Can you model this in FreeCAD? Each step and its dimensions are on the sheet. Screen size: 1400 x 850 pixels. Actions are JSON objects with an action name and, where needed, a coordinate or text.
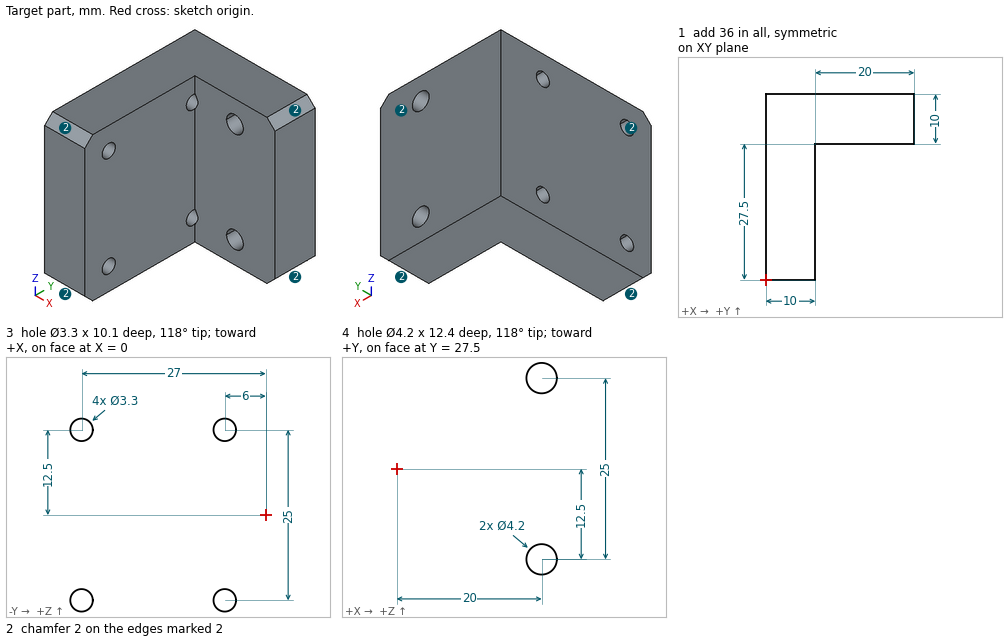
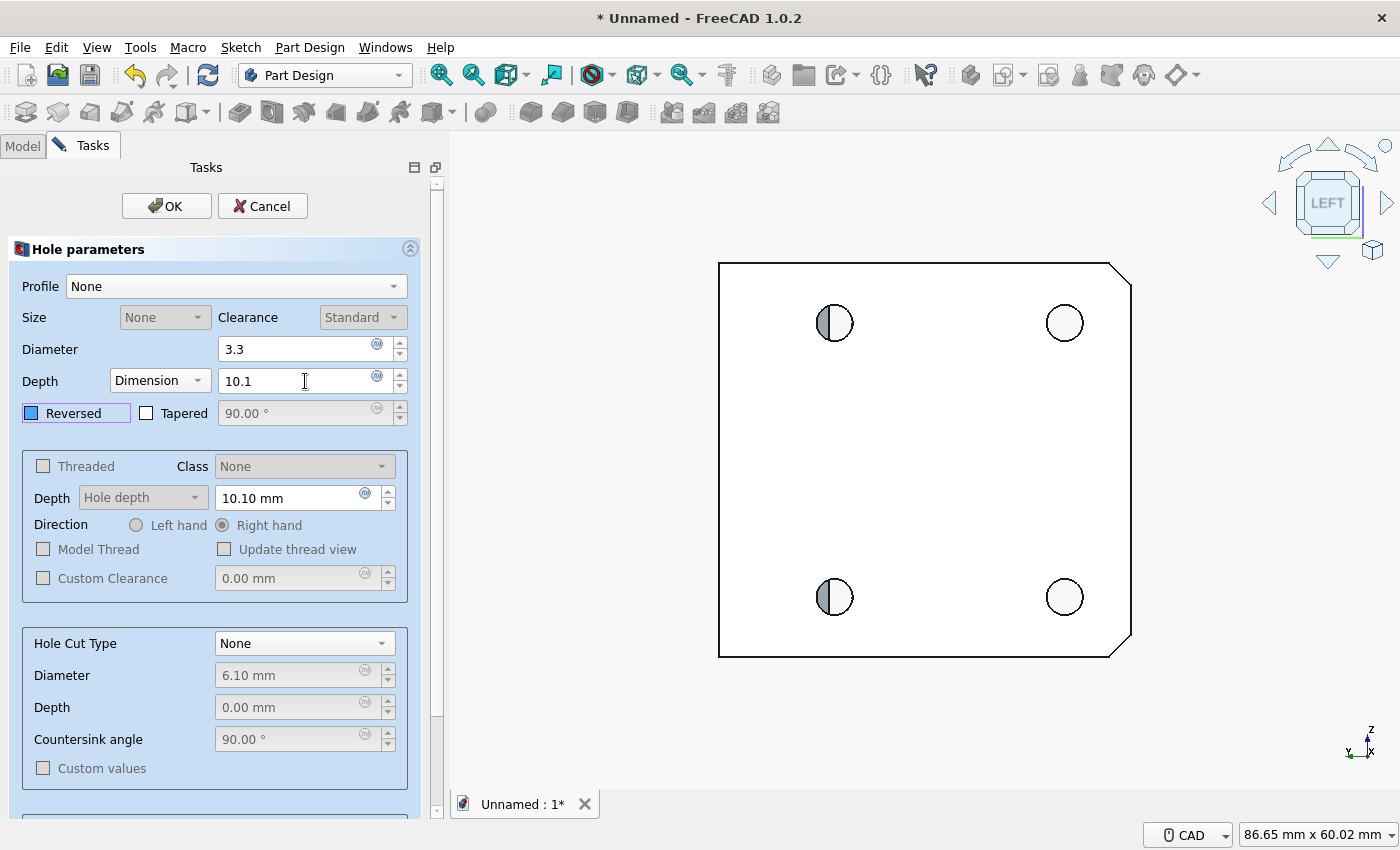
{"action": "left_click", "coordinate": [167, 206]}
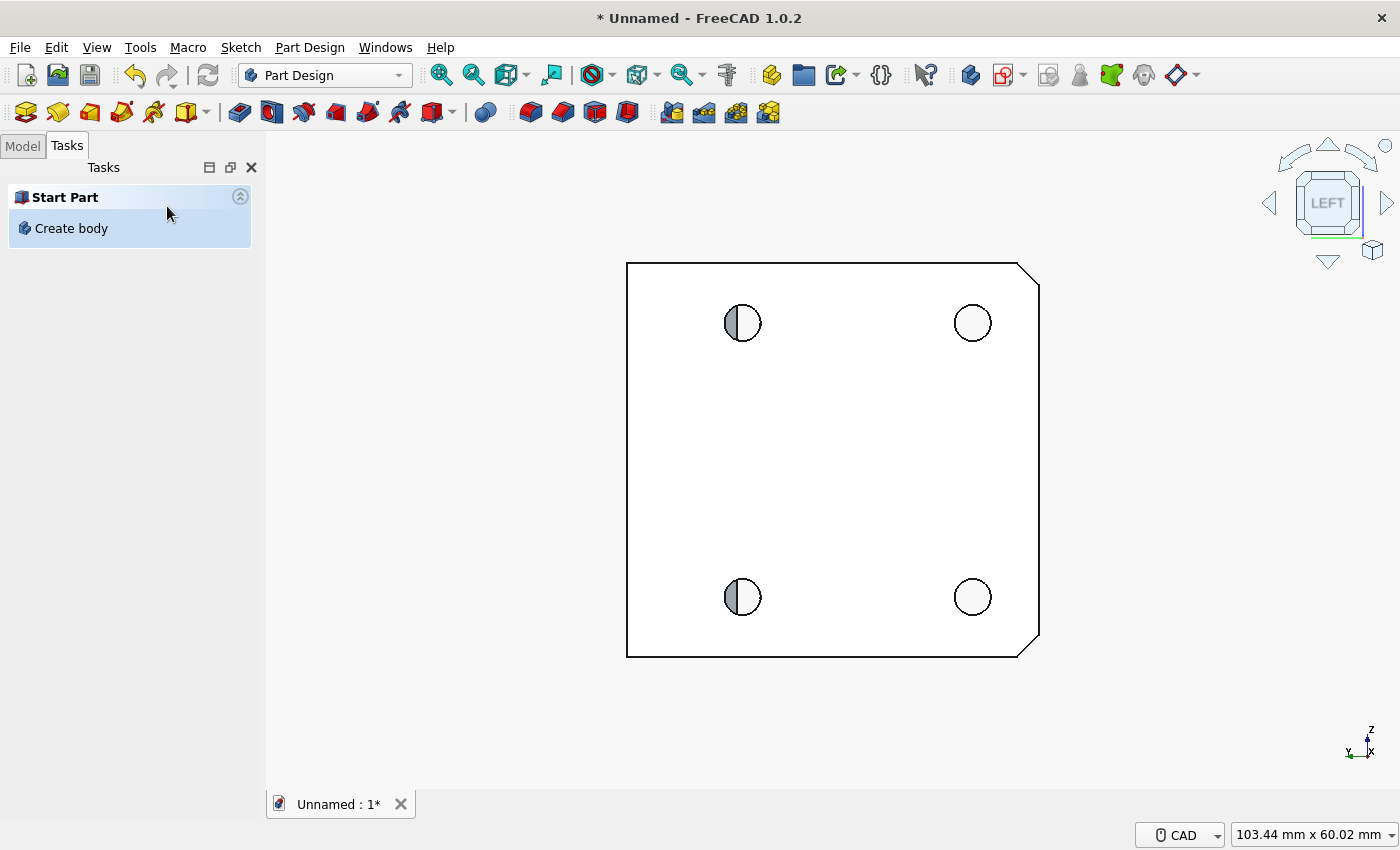
{"action": "key", "text": "0"}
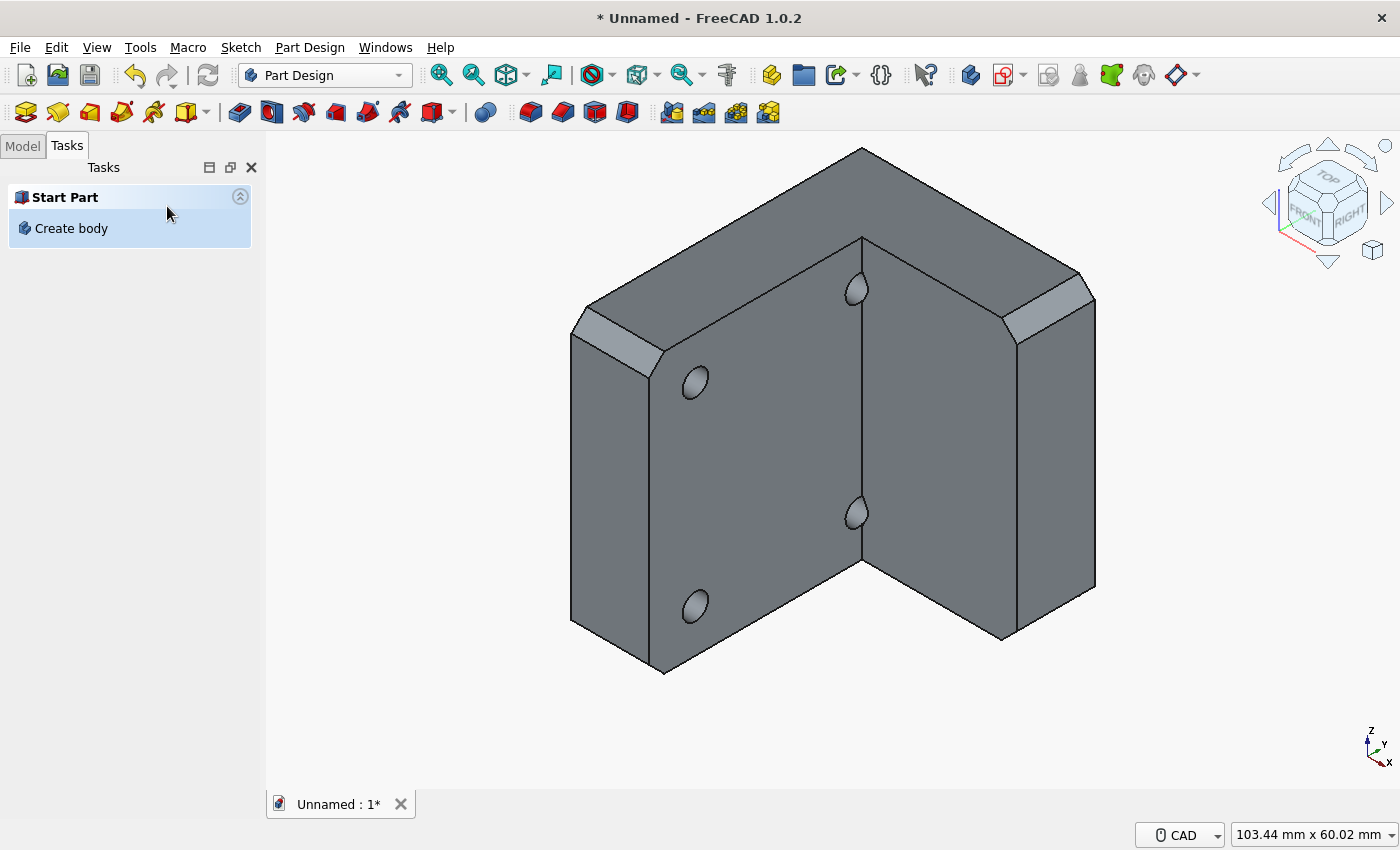
{"action": "left_click", "coordinate": [940, 396]}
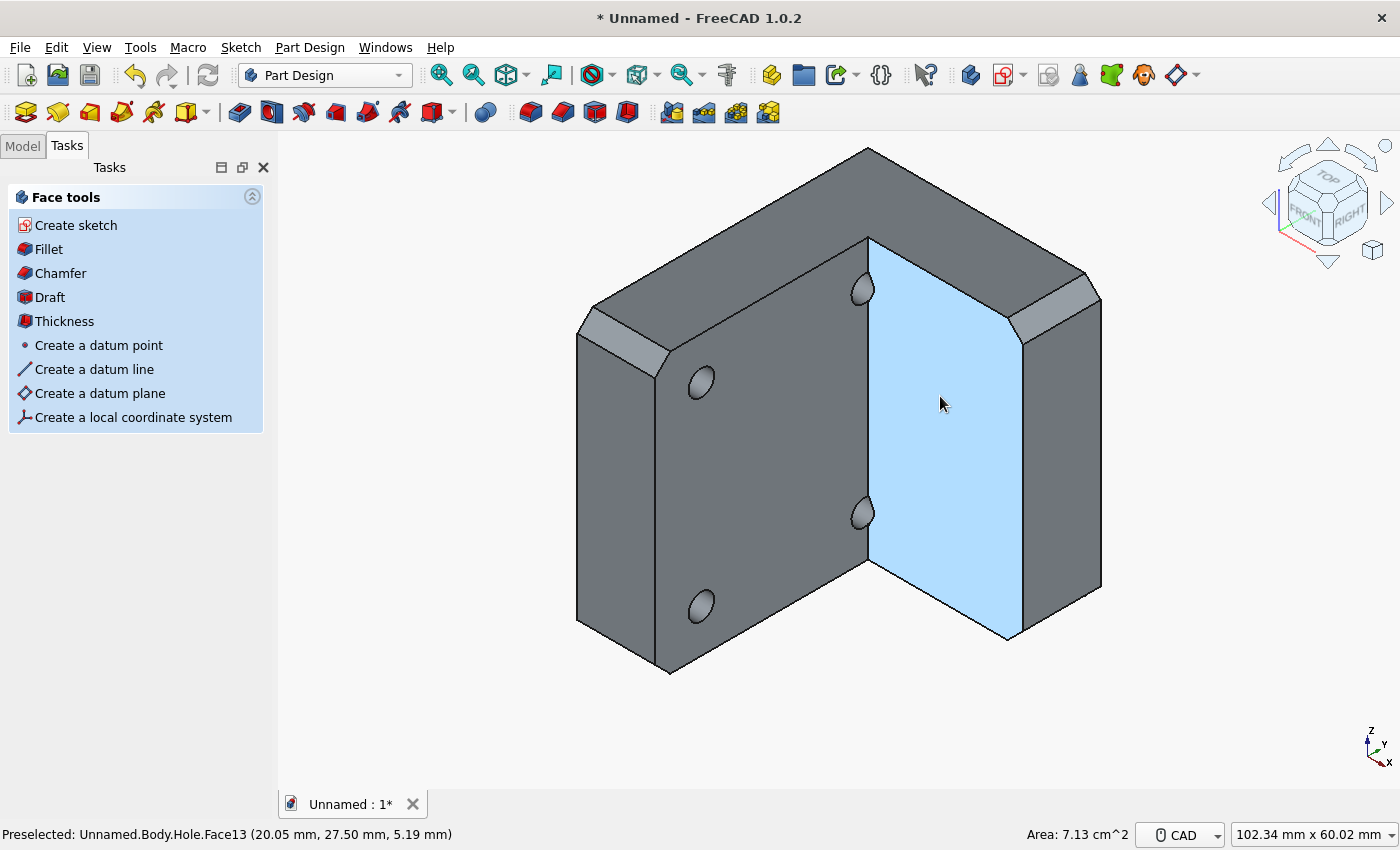
{"action": "left_click", "coordinate": [1004, 76]}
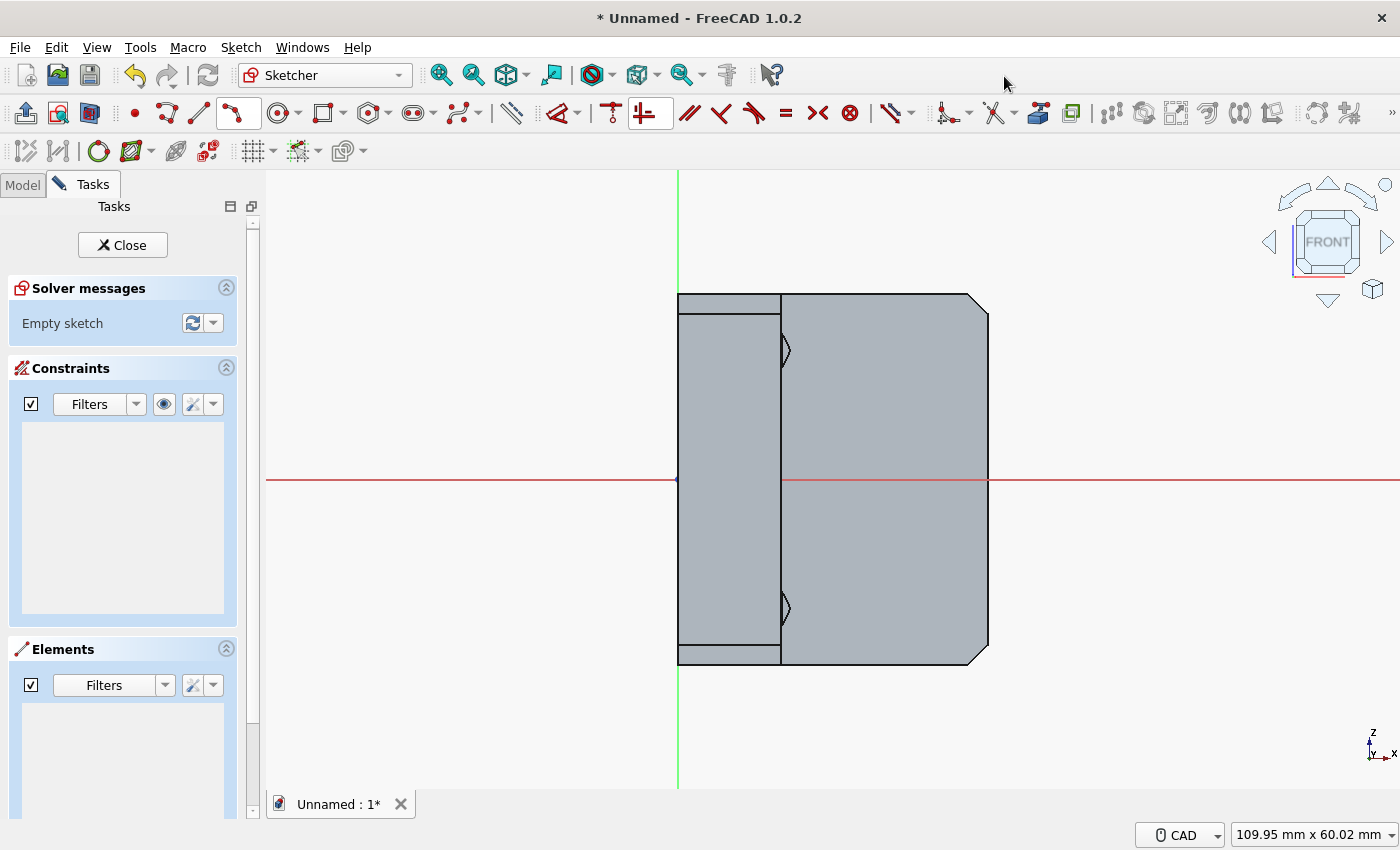
{"action": "key", "text": "g c"}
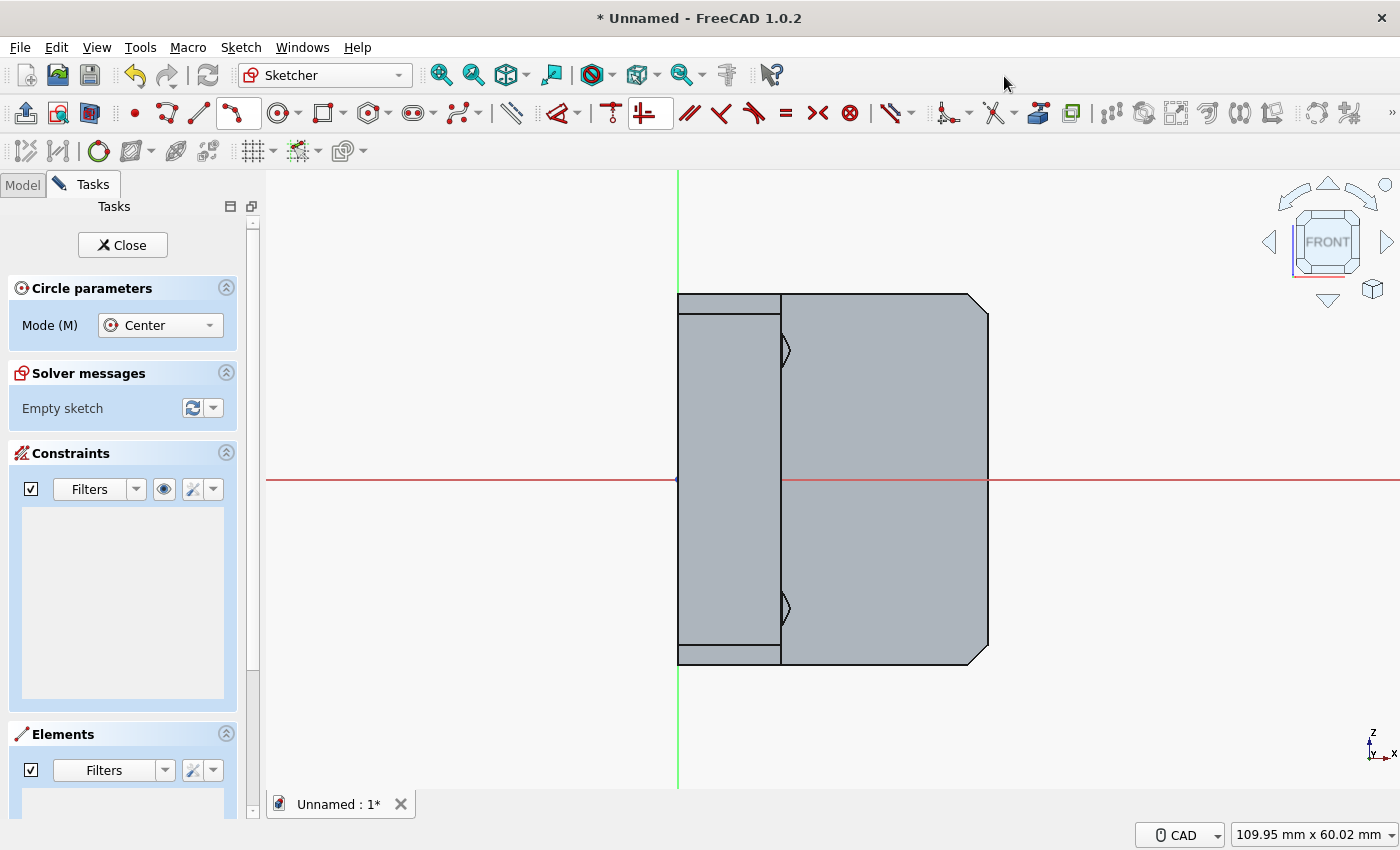
{"action": "left_click", "coordinate": [885, 608]}
{"action": "left_click", "coordinate": [900, 593]}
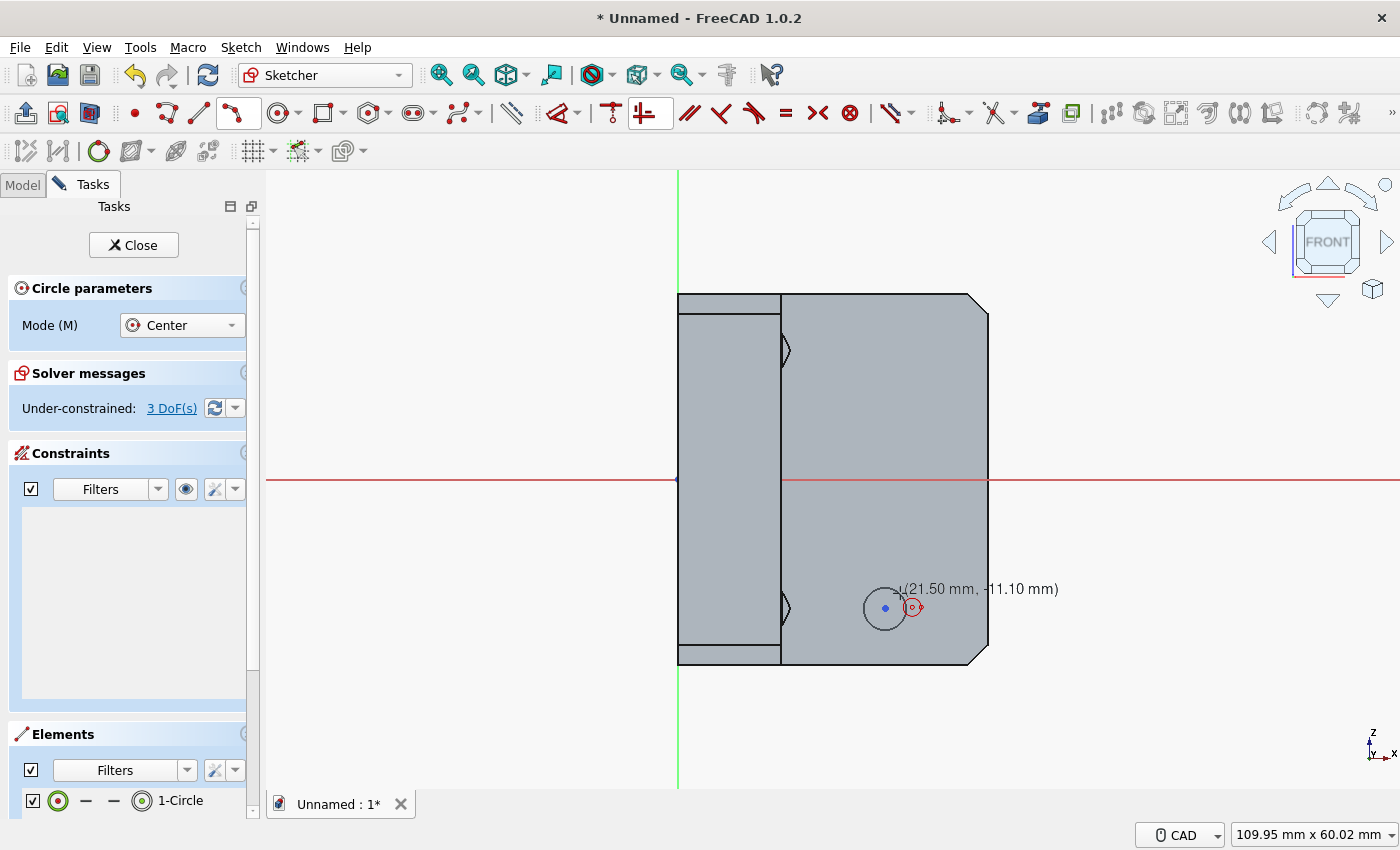
{"action": "left_click", "coordinate": [885, 351]}
{"action": "left_click", "coordinate": [900, 335]}
{"action": "key", "text": "Escape"}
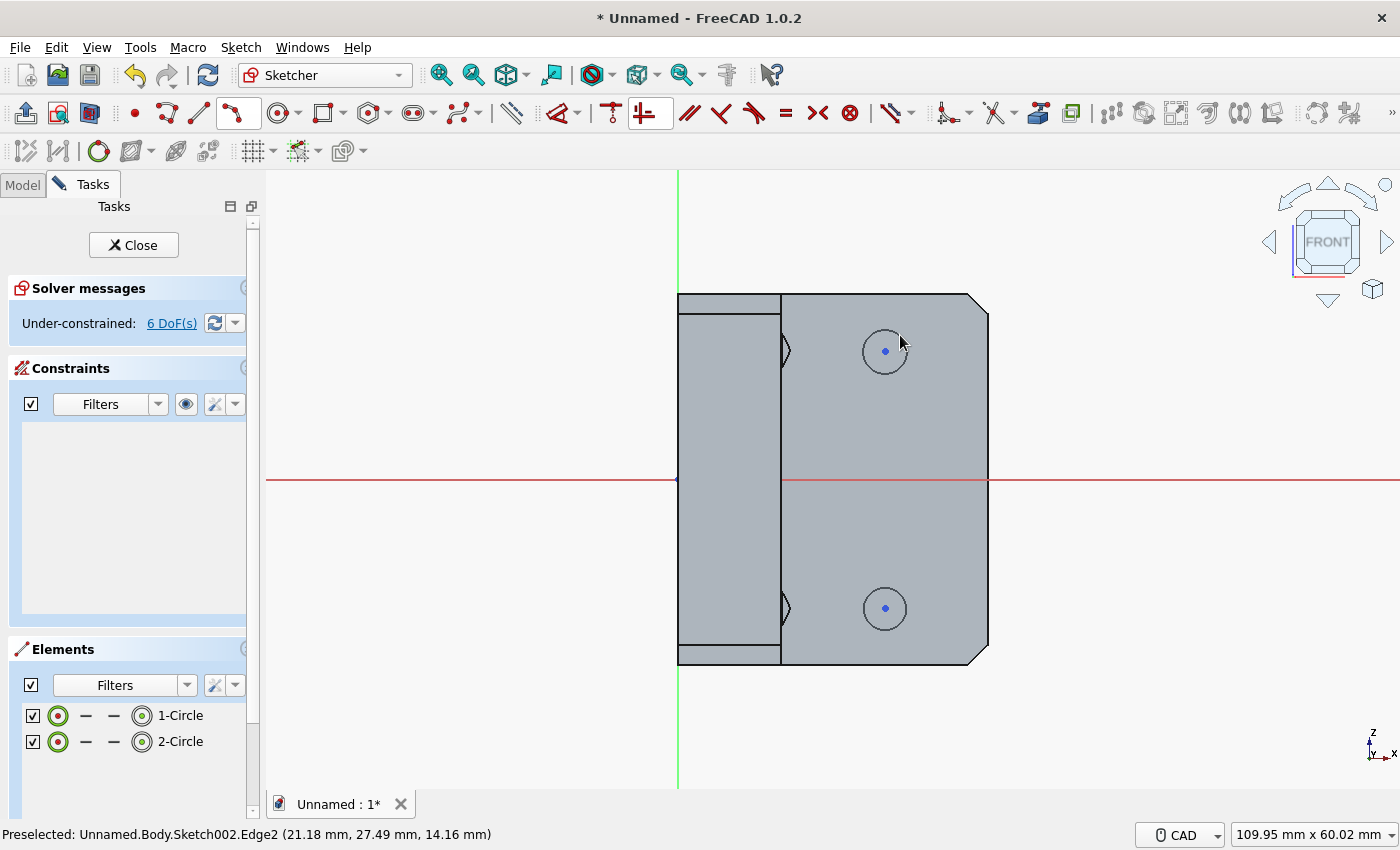
{"action": "left_click", "coordinate": [900, 594]}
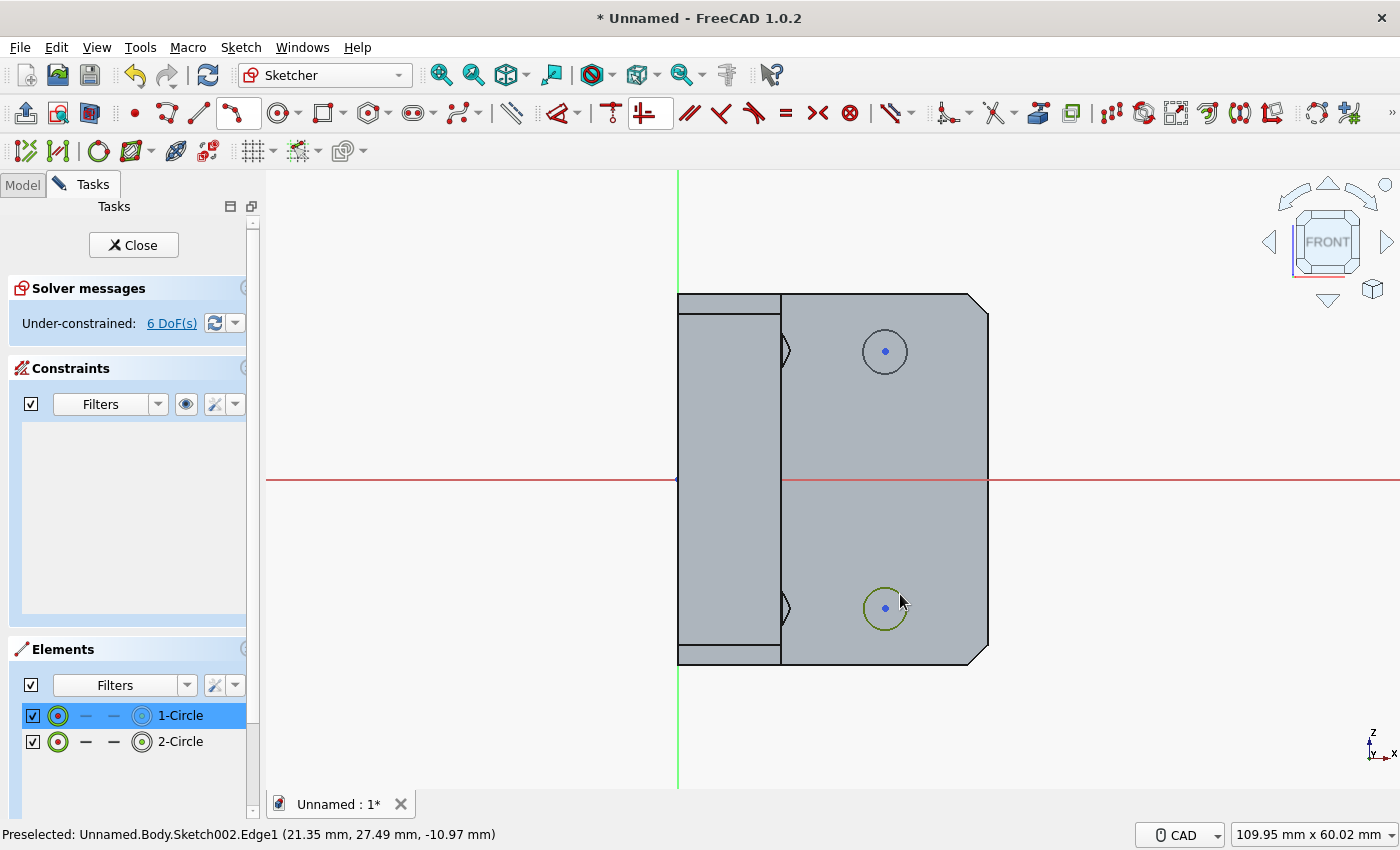
{"action": "left_click", "coordinate": [900, 336]}